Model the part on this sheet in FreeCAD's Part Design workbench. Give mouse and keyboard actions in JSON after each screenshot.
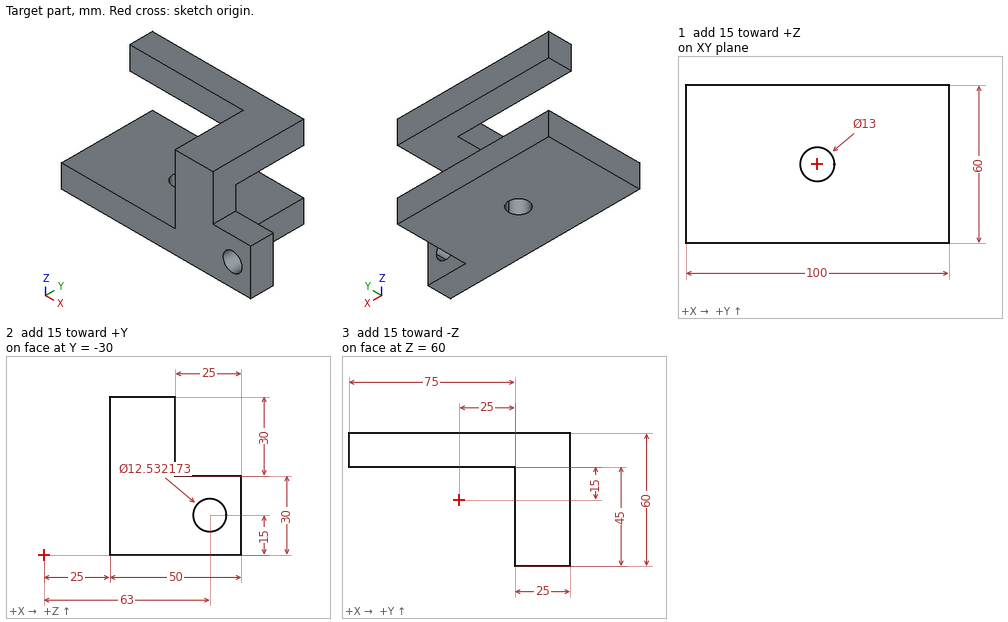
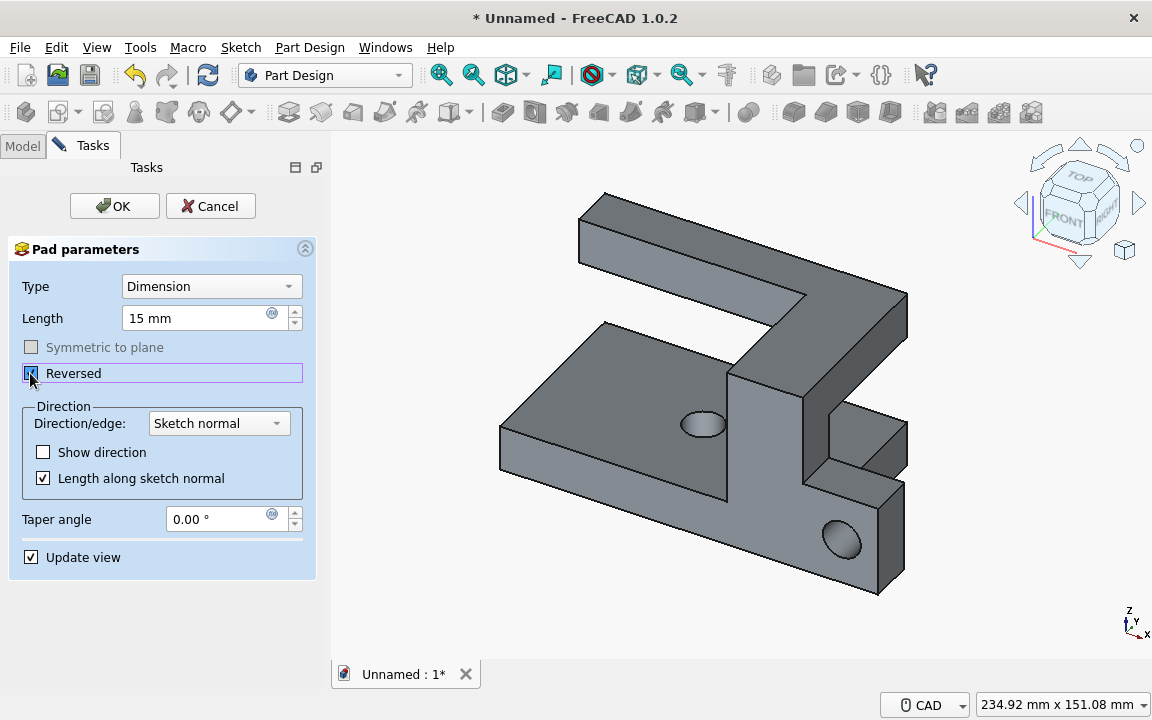
{"action": "left_click", "coordinate": [115, 206]}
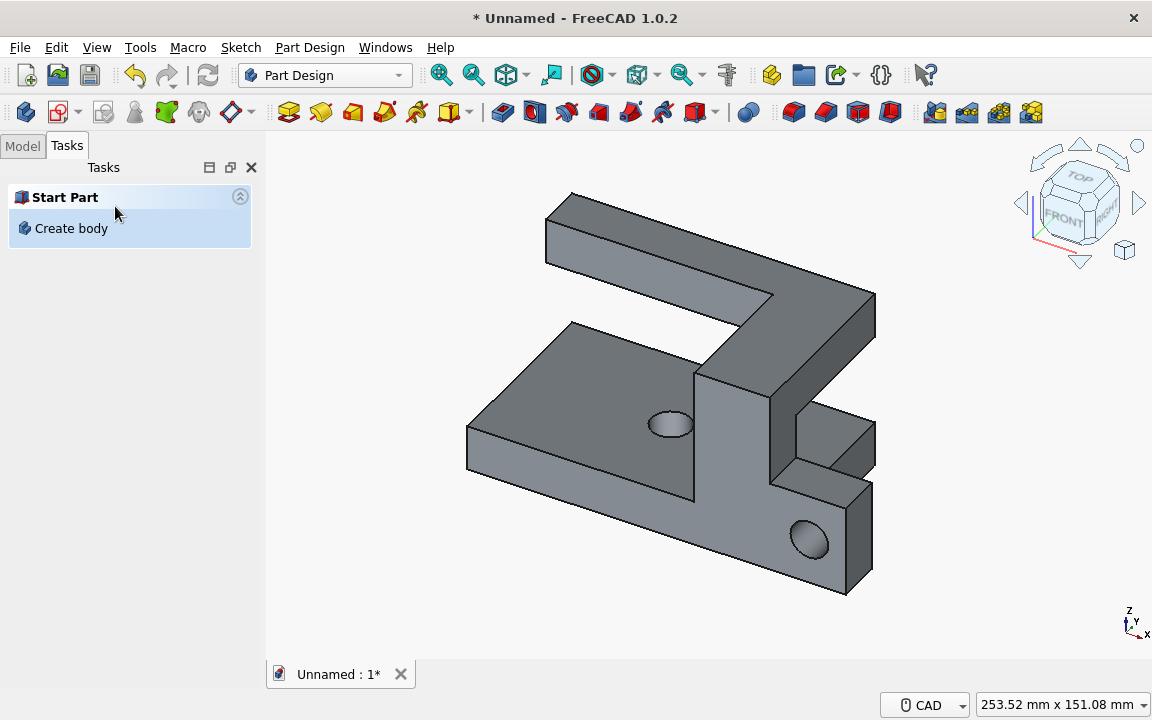
{"action": "key", "text": "0"}